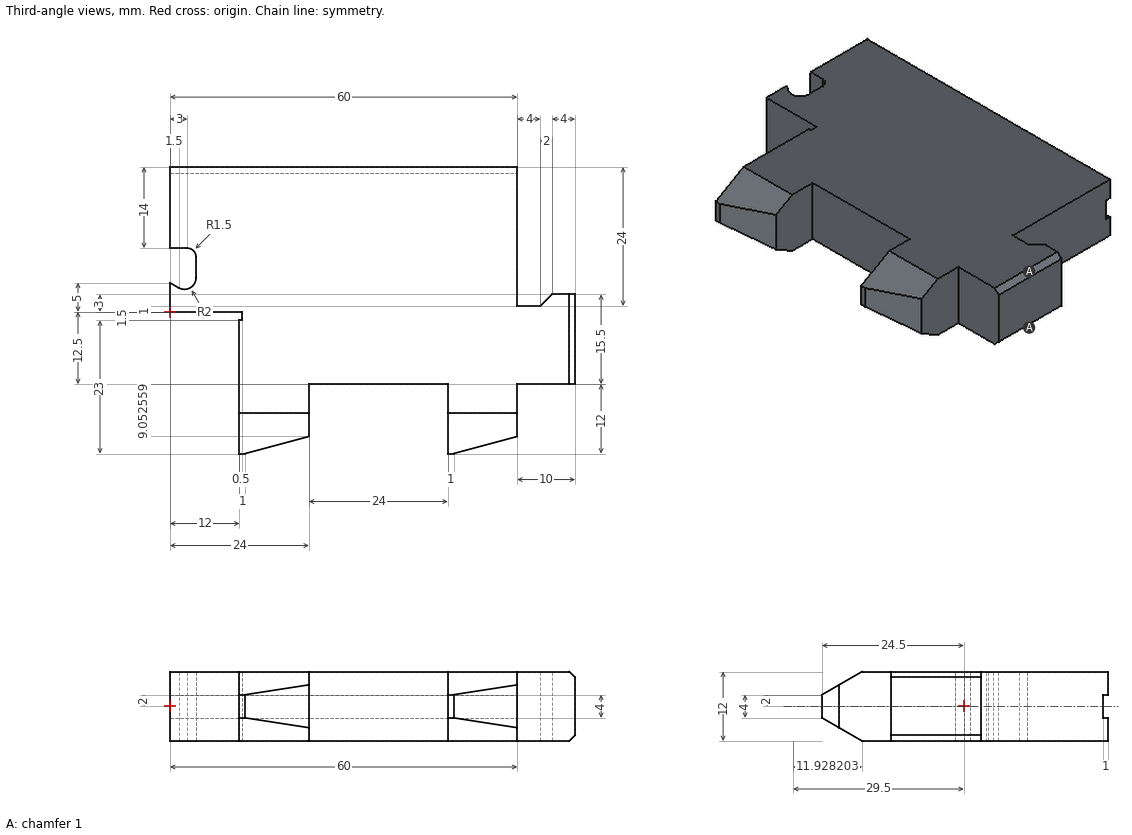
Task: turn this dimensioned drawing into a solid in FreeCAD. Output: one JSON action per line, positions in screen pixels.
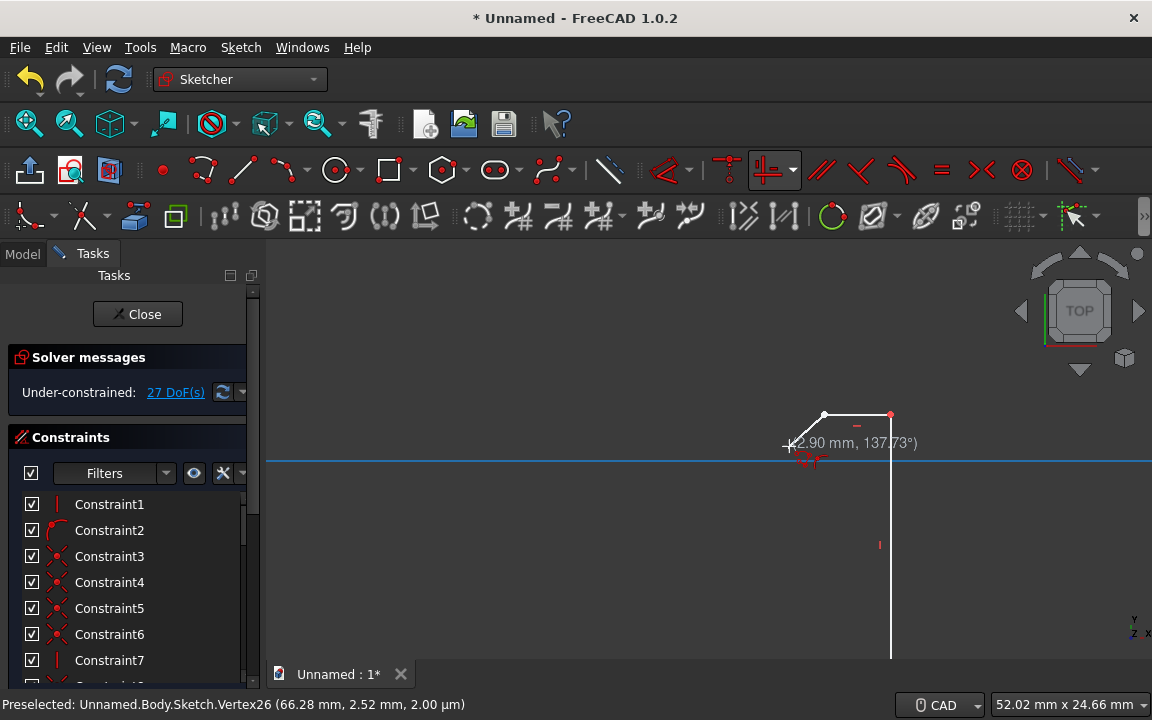
{"action": "left_click", "coordinate": [789, 444]}
{"action": "left_click", "coordinate": [721, 444]}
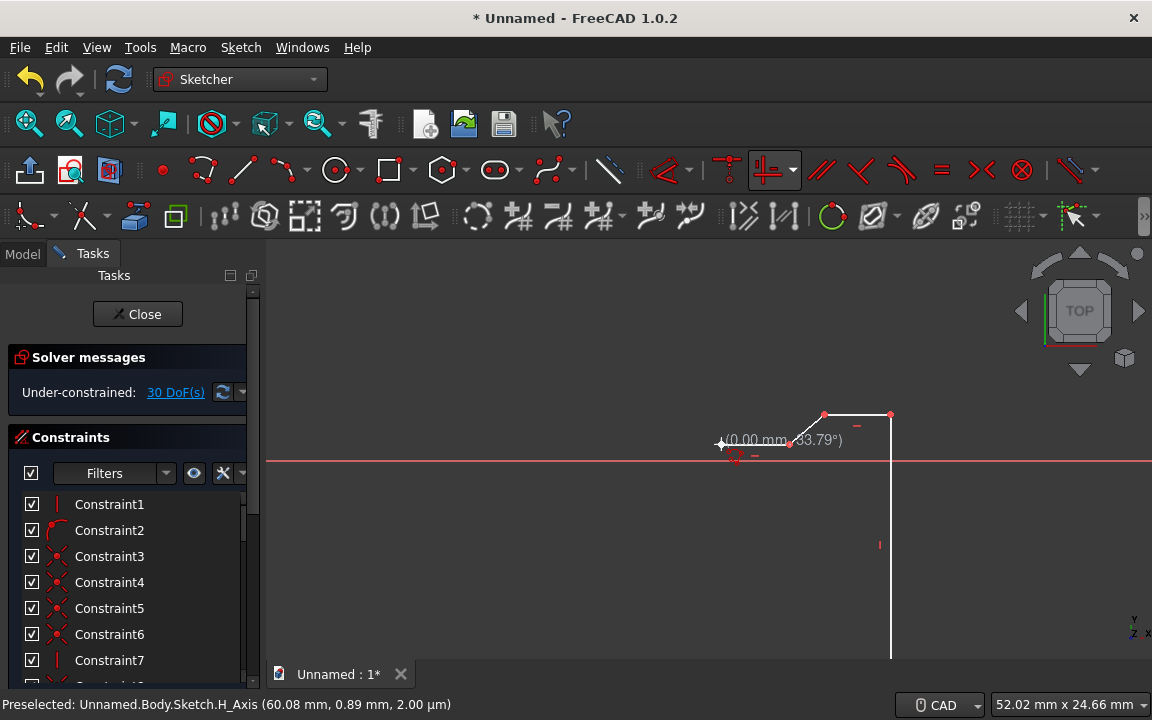
{"action": "scroll", "coordinate": [790, 446], "scroll_direction": "down", "scroll_amount": 6}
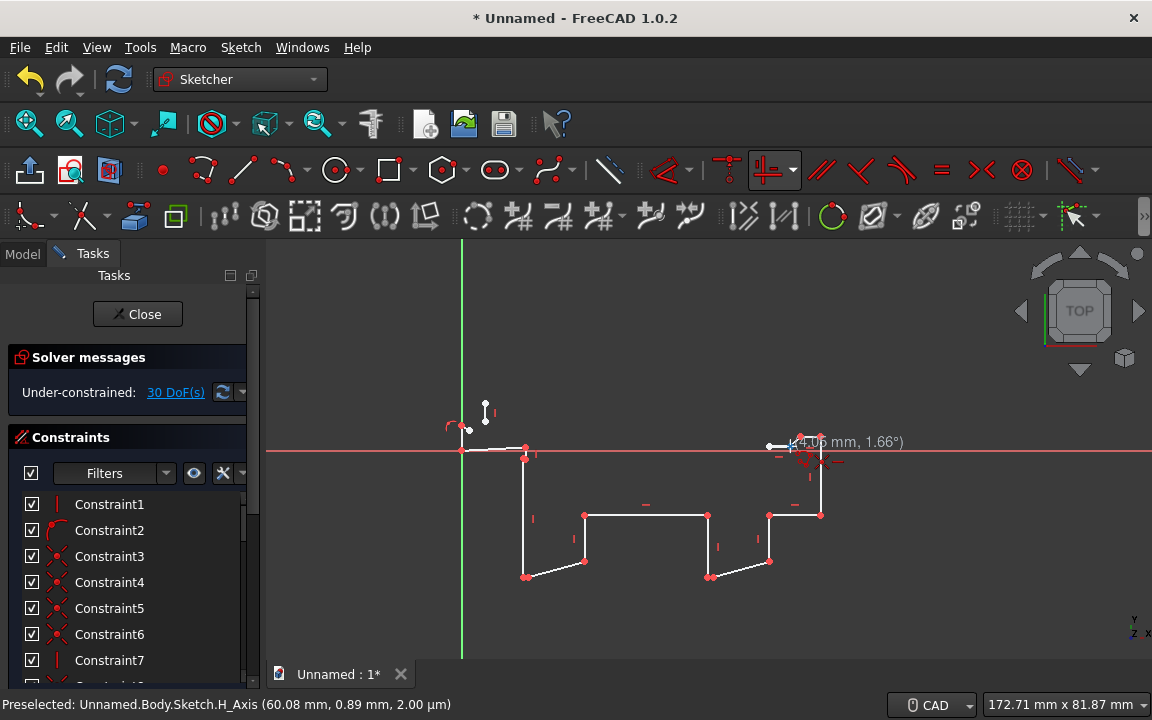
{"action": "left_click", "coordinate": [770, 323]}
{"action": "left_click", "coordinate": [462, 323]}
{"action": "left_click", "coordinate": [471, 394]}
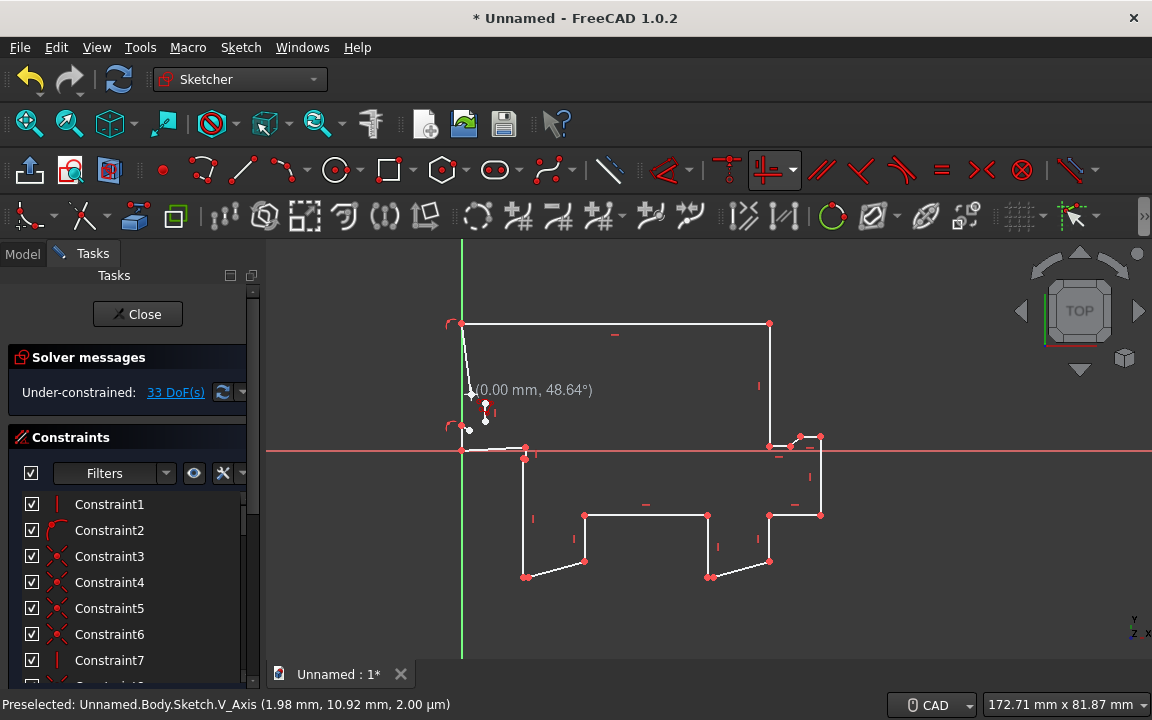
{"action": "scroll", "coordinate": [477, 394], "scroll_direction": "up", "scroll_amount": 2}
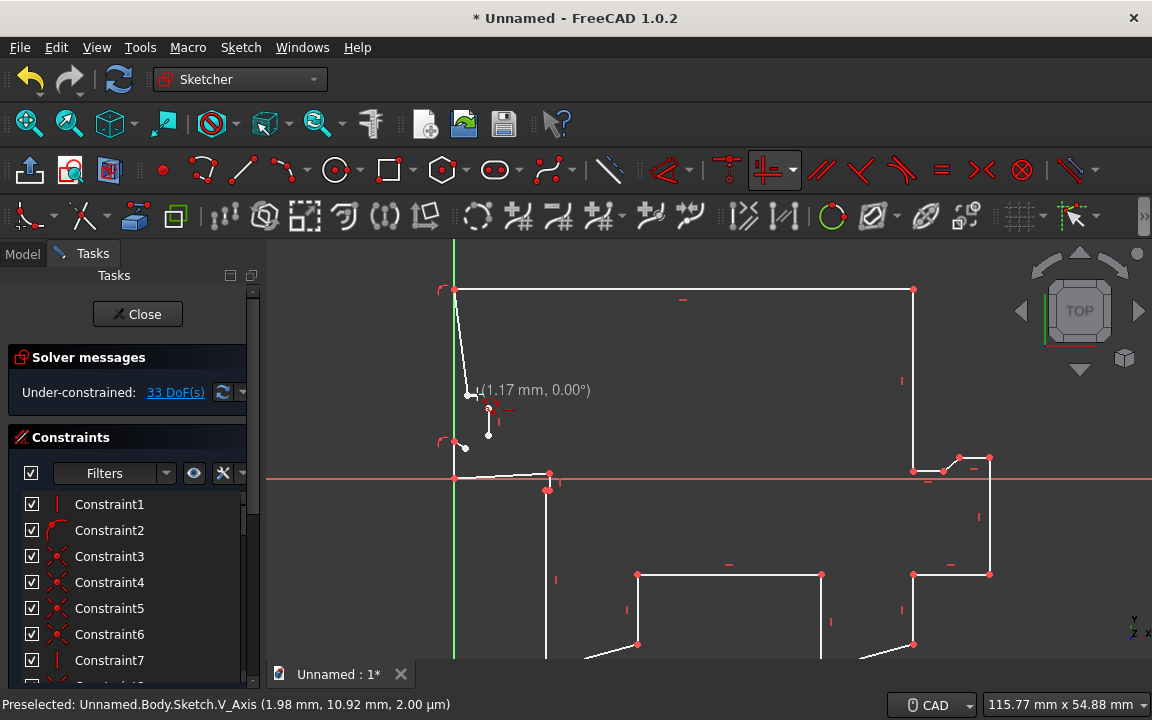
{"action": "left_click", "coordinate": [477, 394]}
{"action": "right_click", "coordinate": [477, 394]}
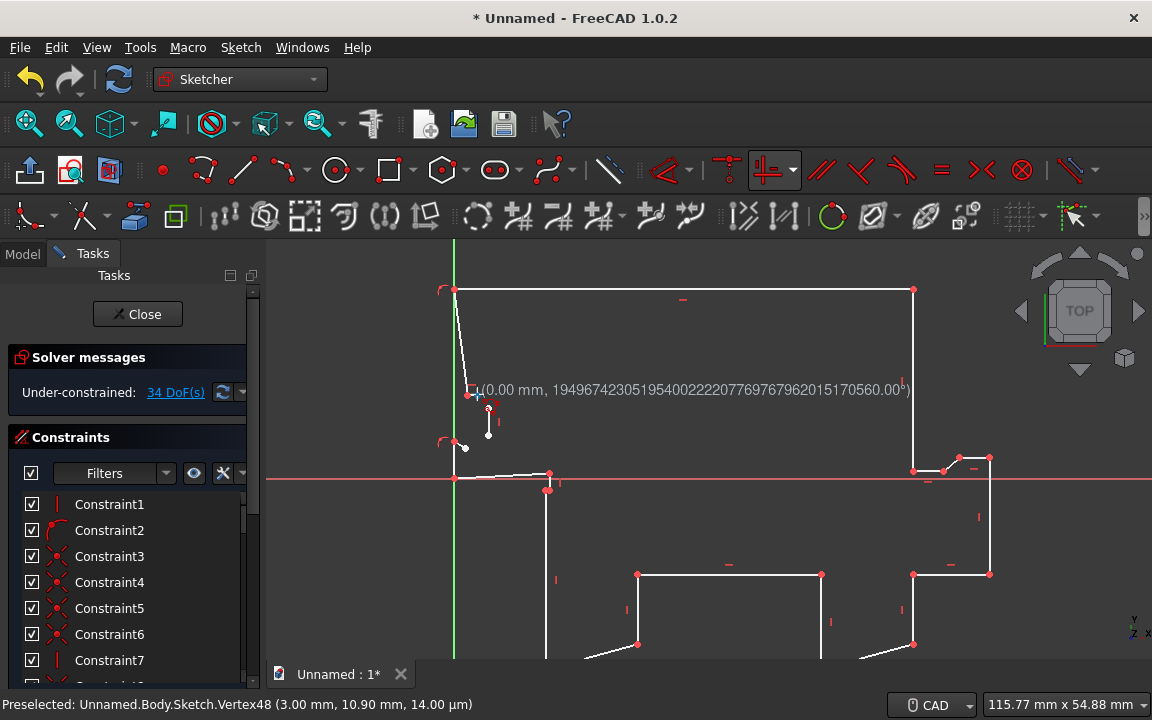
{"action": "left_click", "coordinate": [284, 170]}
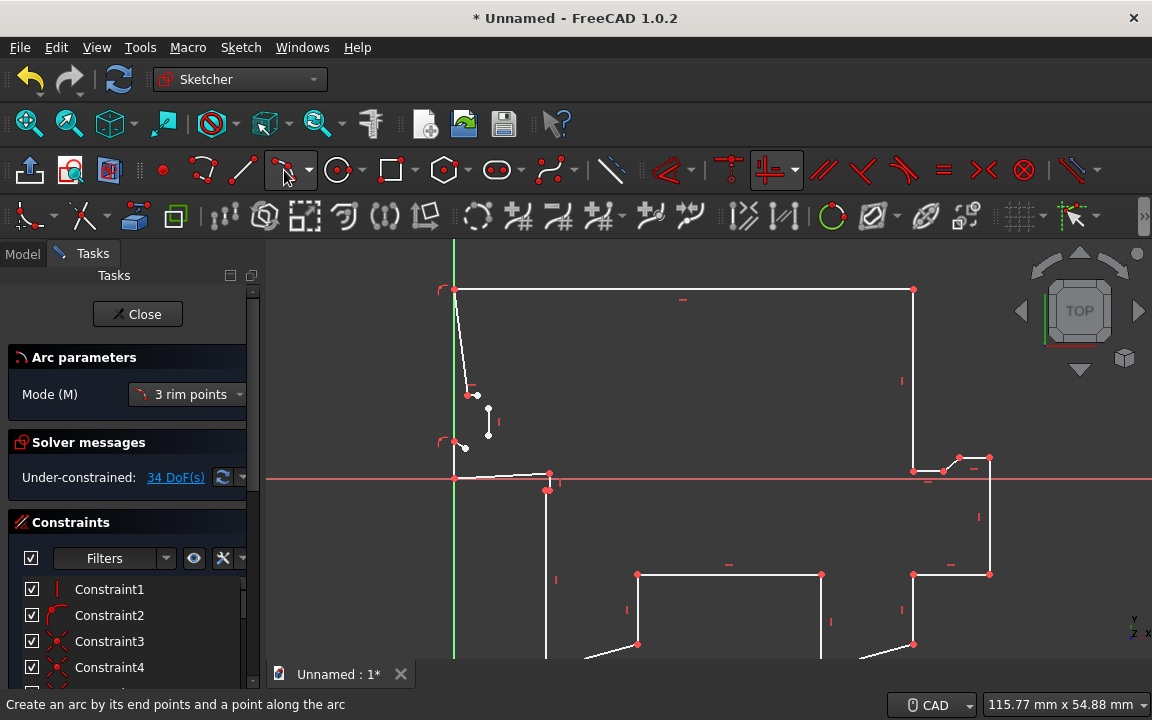
{"action": "left_click", "coordinate": [489, 435]}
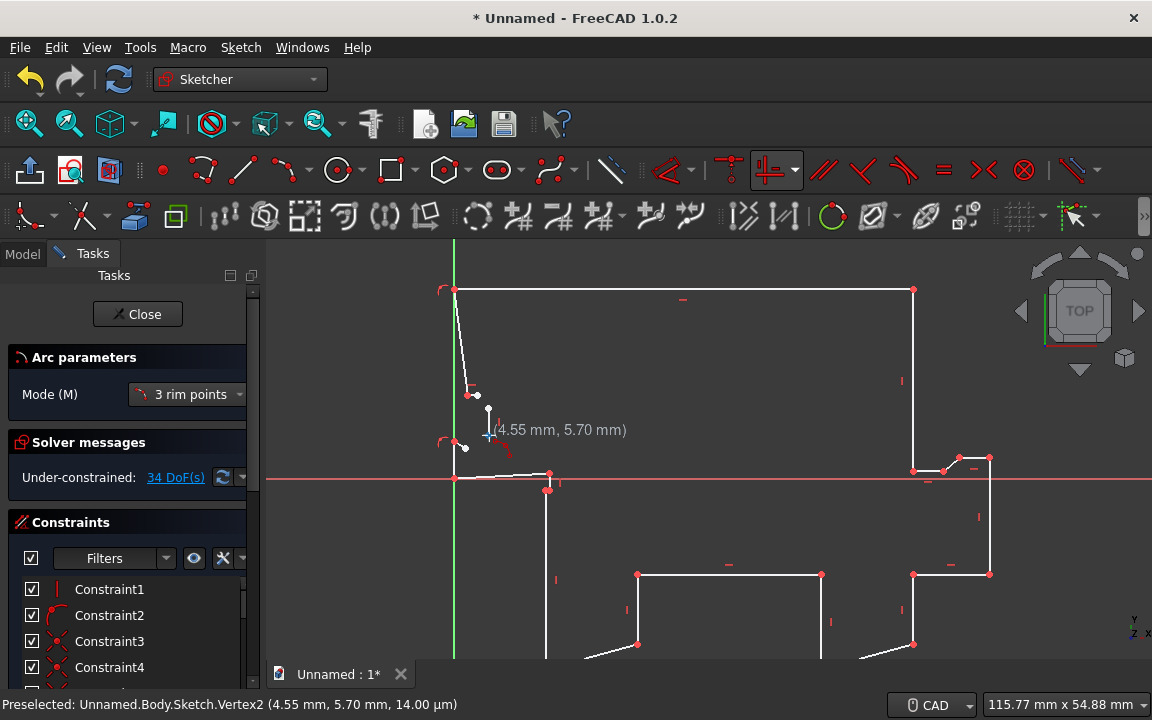
{"action": "scroll", "coordinate": [466, 447], "scroll_direction": "up", "scroll_amount": 5}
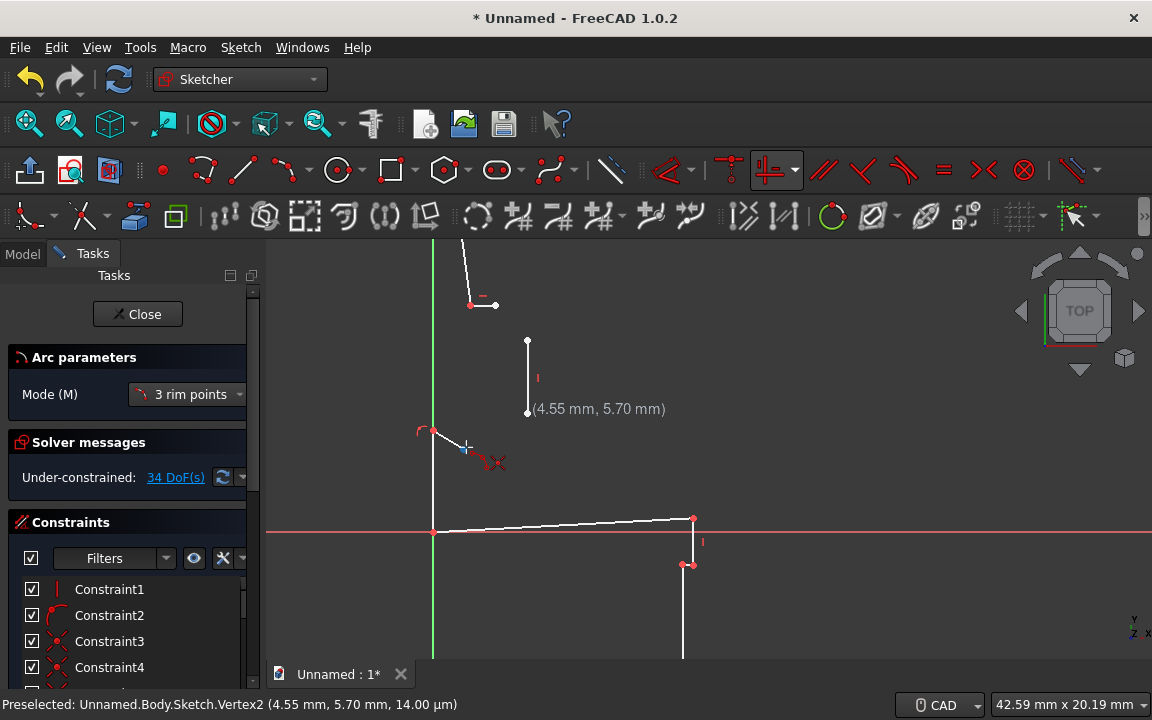
{"action": "left_click", "coordinate": [464, 449]}
{"action": "left_click", "coordinate": [506, 446]}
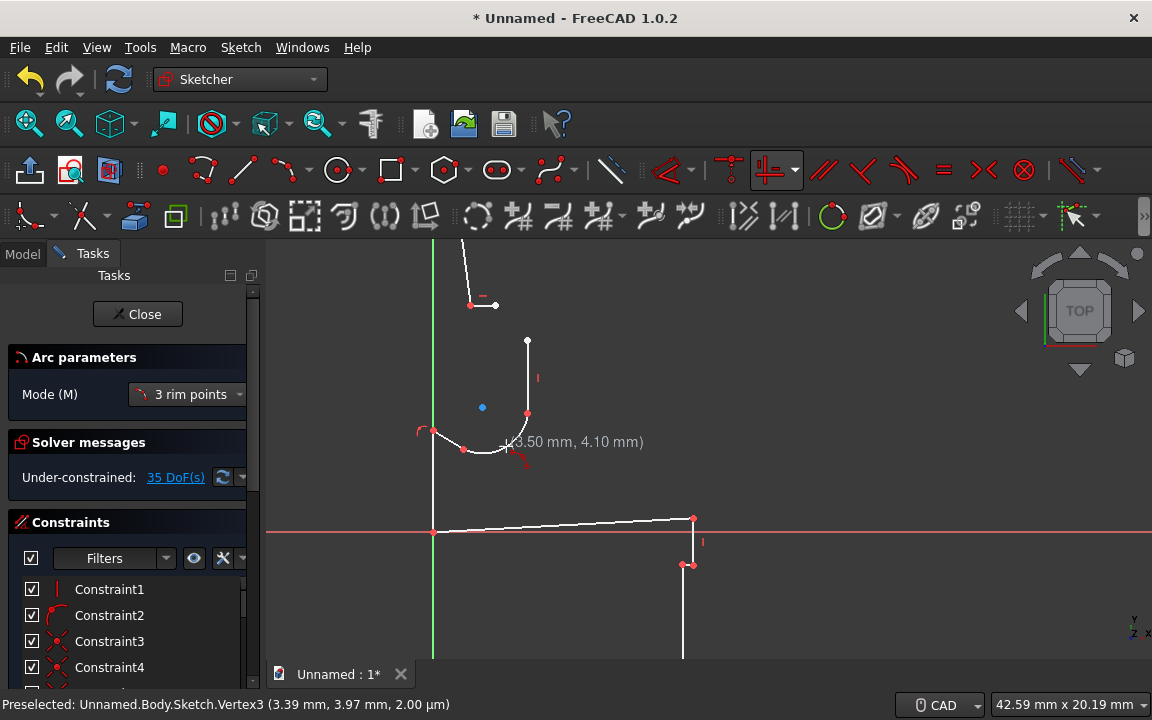
{"action": "left_click", "coordinate": [496, 306]}
{"action": "left_click", "coordinate": [528, 341]}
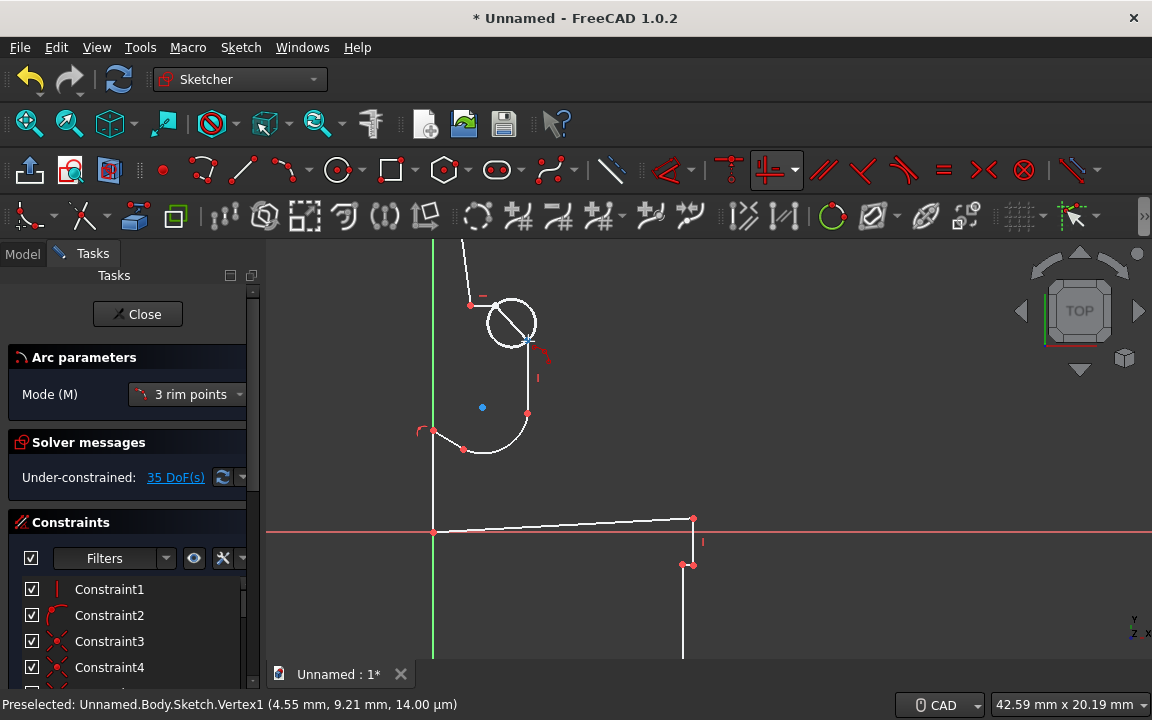
{"action": "scroll", "coordinate": [518, 313], "scroll_direction": "up", "scroll_amount": 3}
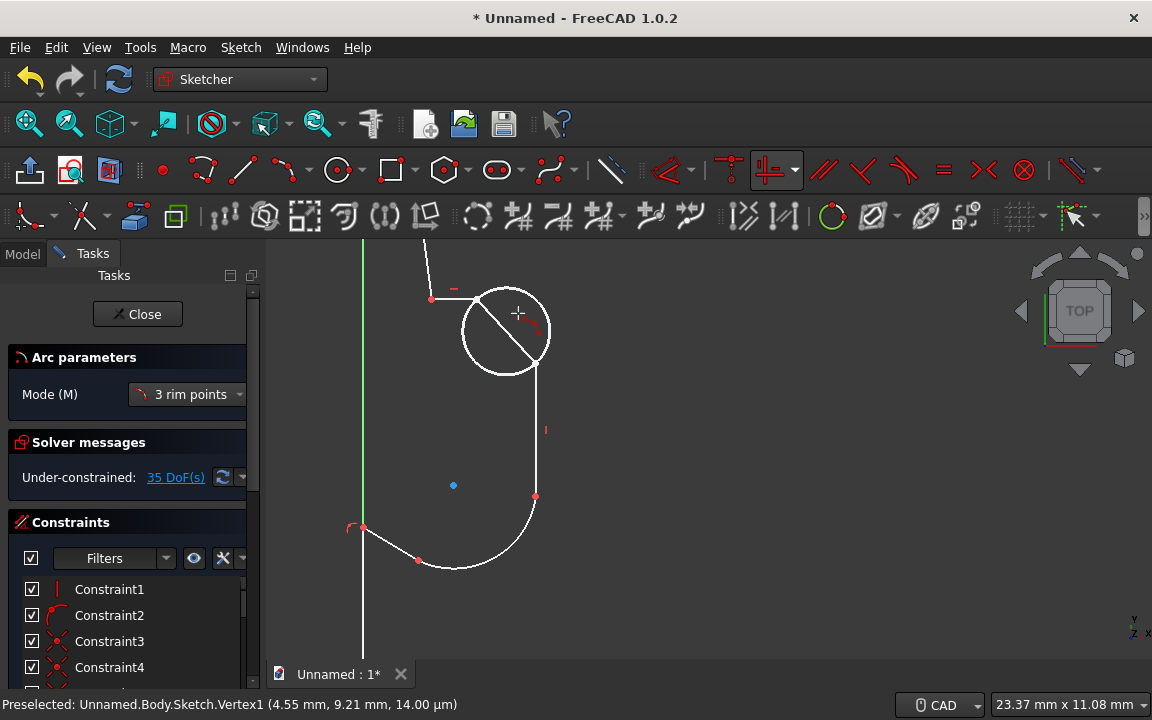
{"action": "left_click", "coordinate": [517, 312]}
{"action": "key", "text": "Escape"}